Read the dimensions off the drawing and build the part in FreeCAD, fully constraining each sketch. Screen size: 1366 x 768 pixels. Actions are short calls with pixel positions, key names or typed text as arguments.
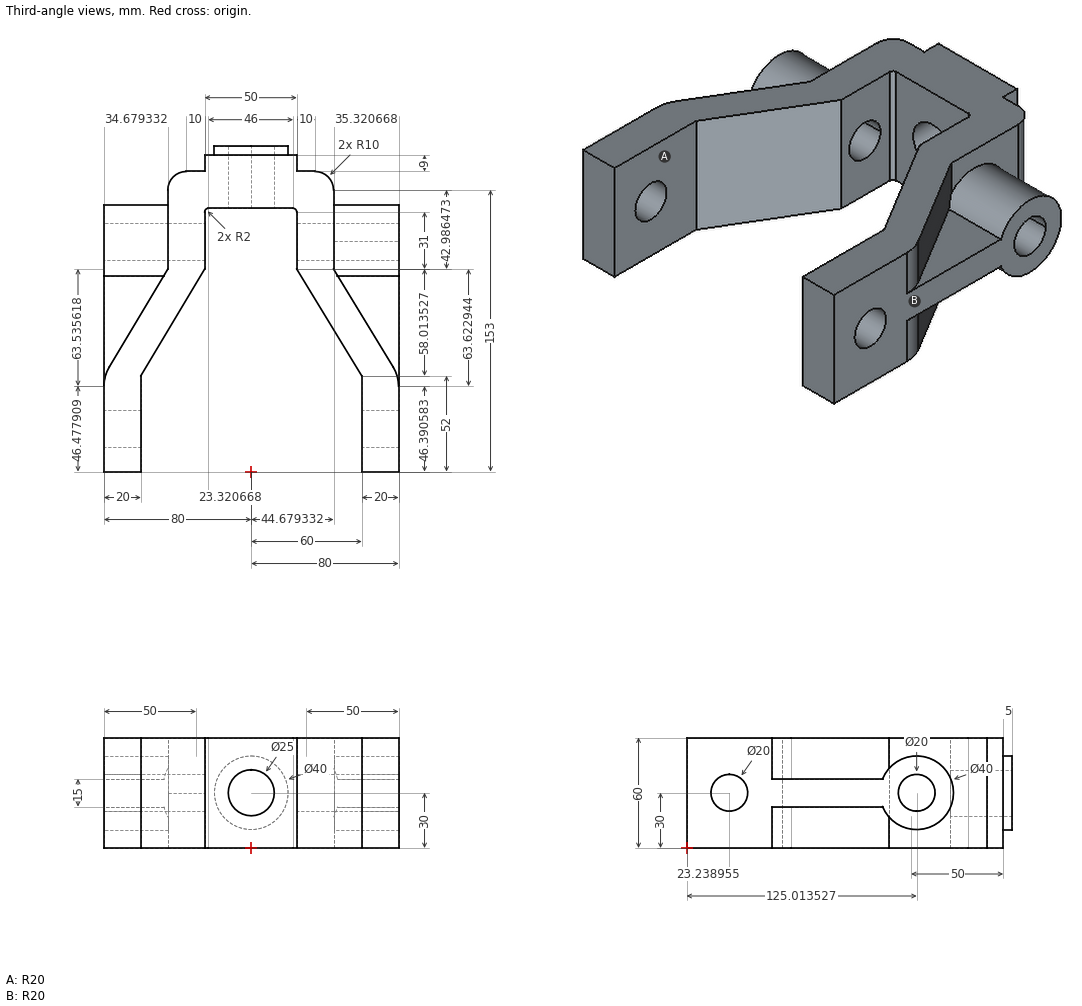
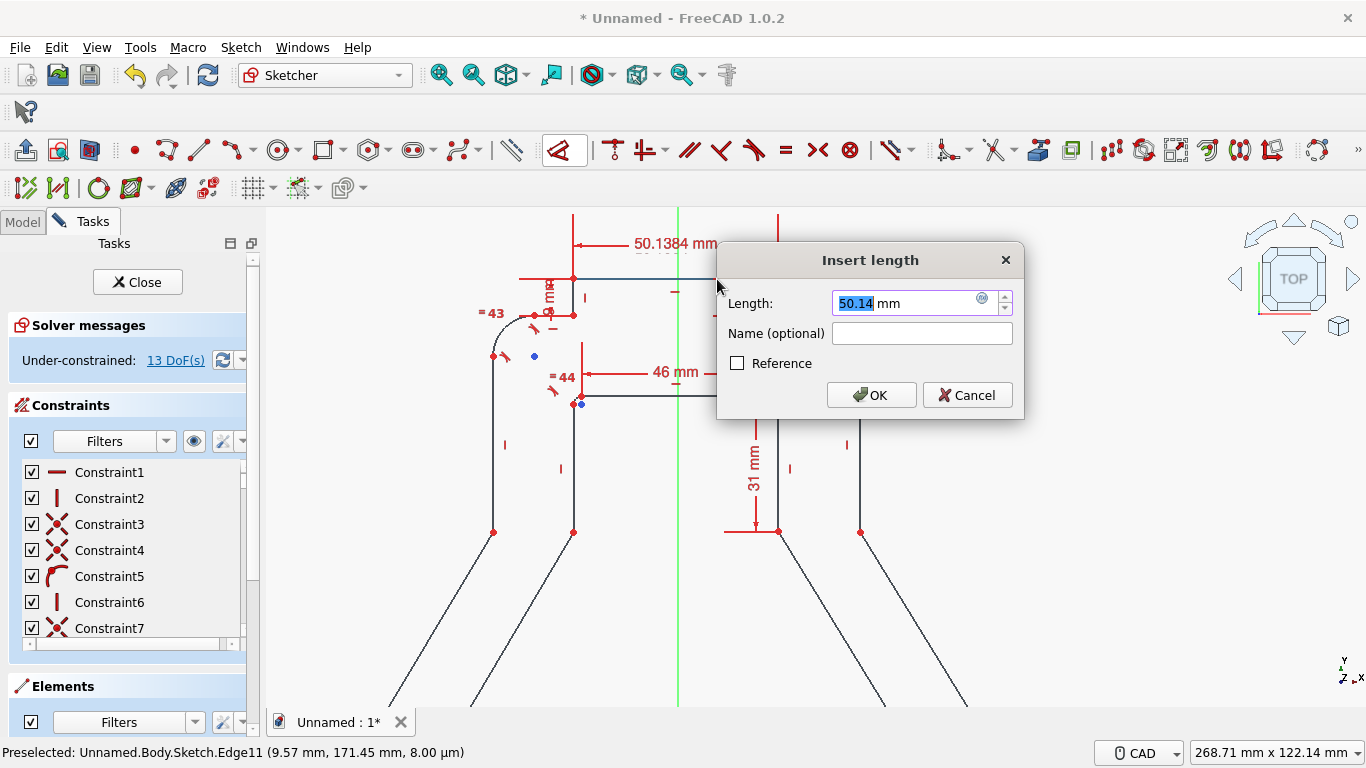
text(50)
key(Return)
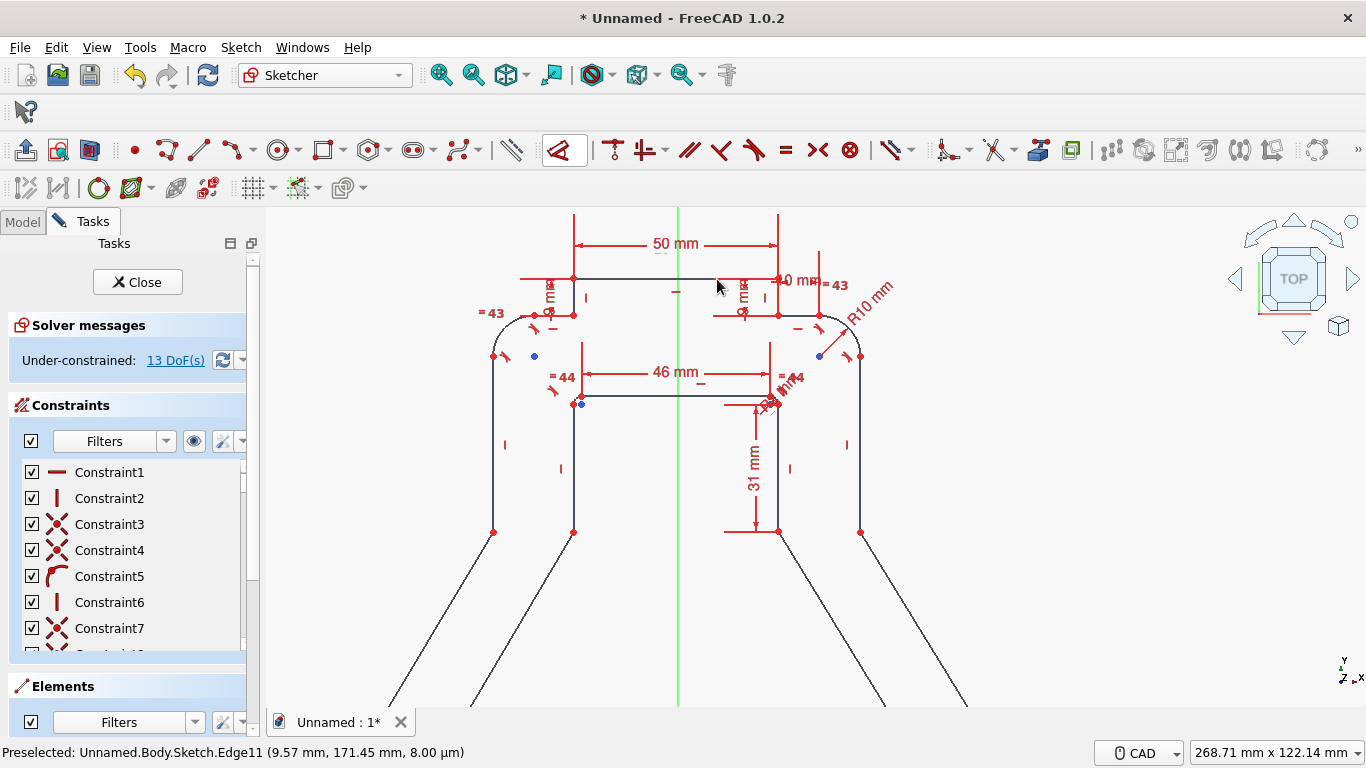
click(562, 316)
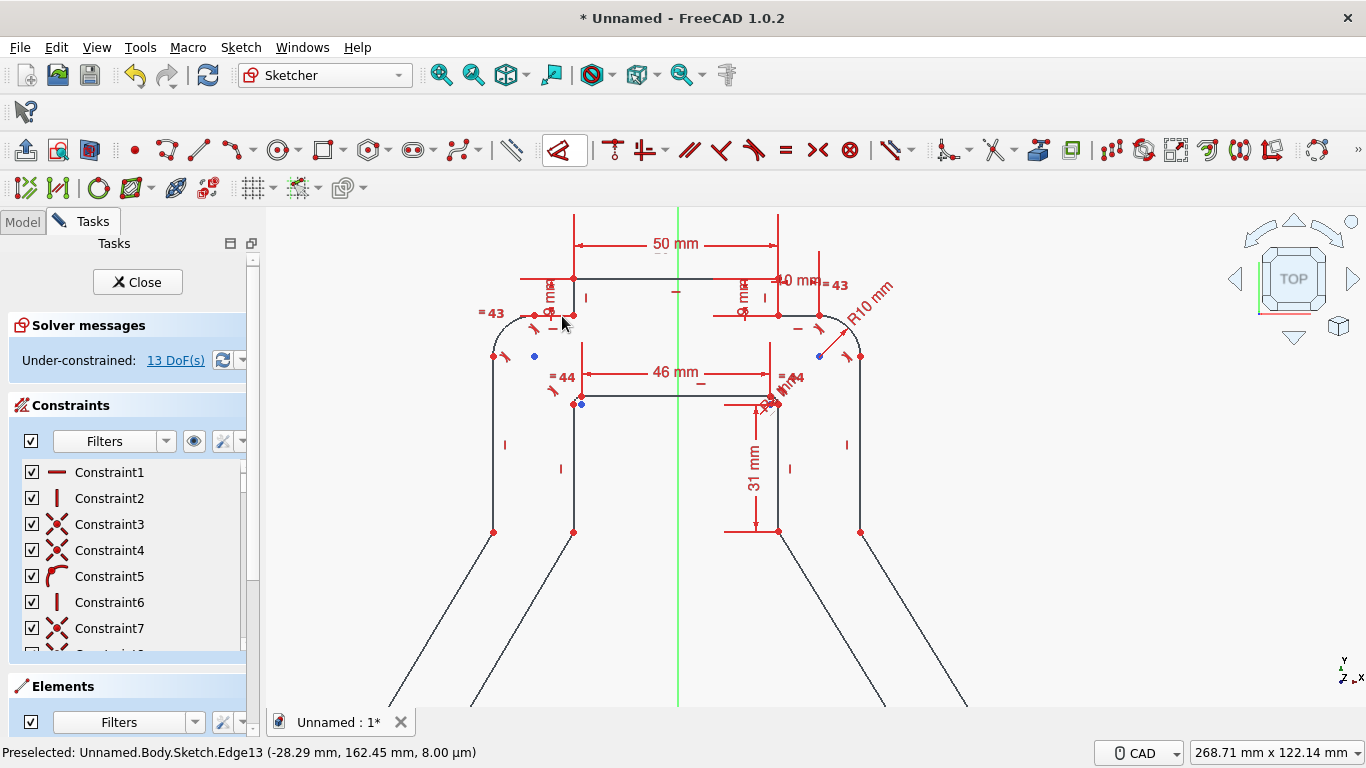
key(l)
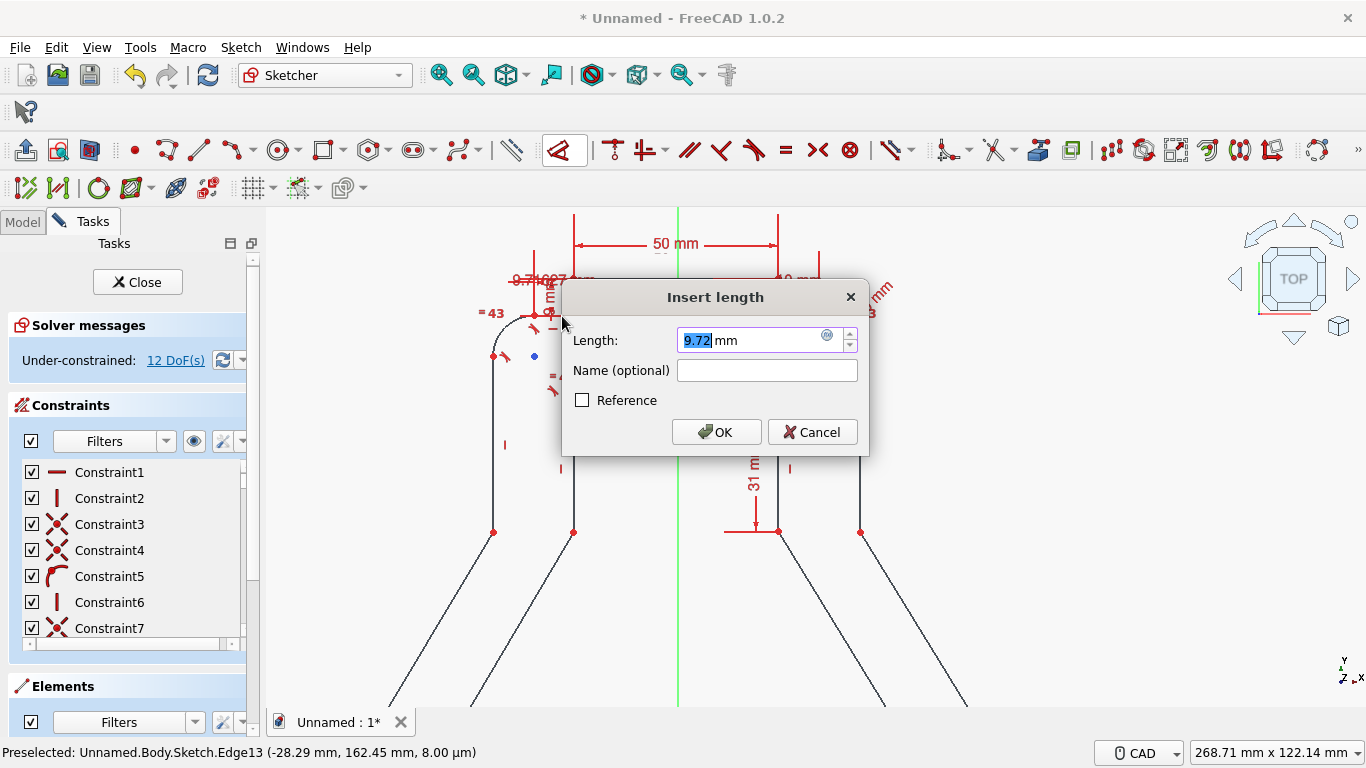
text(10)
key(Return)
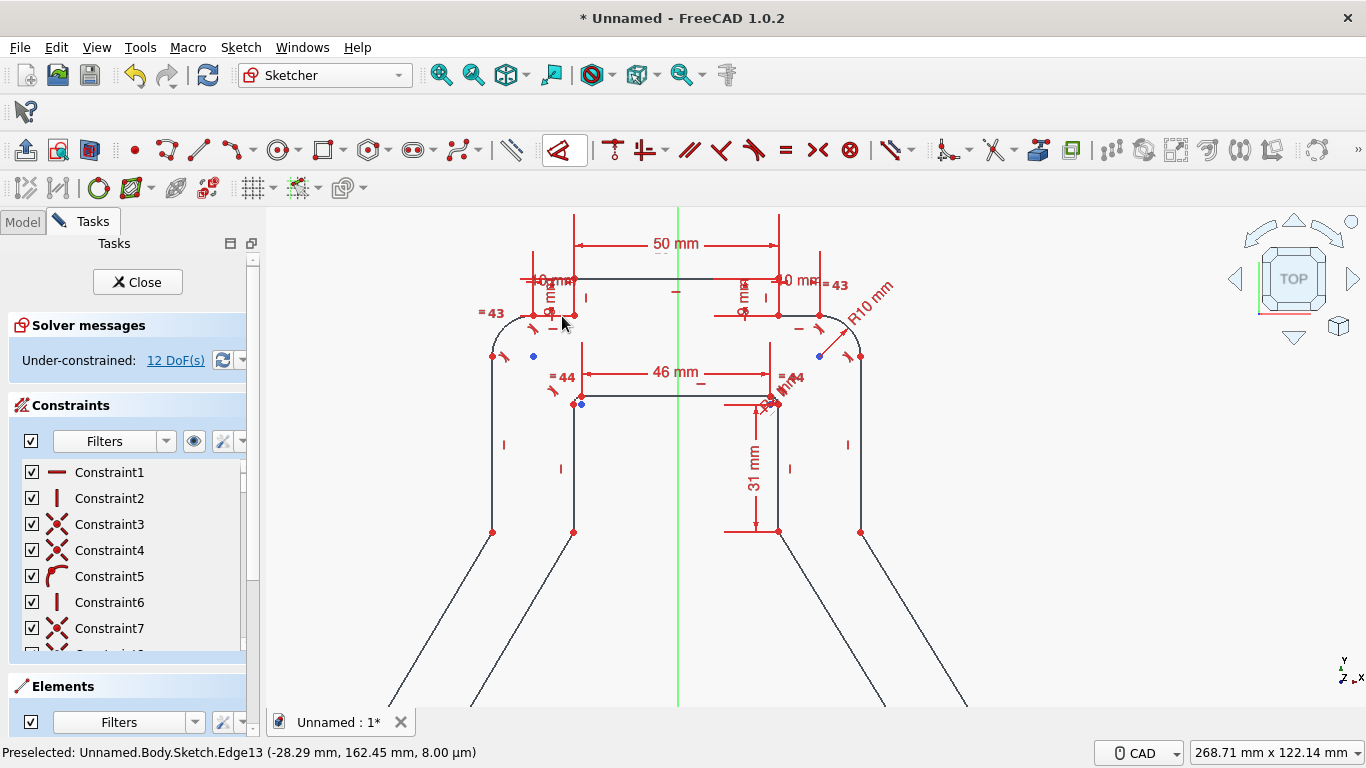
scroll(804, 317, down, 4)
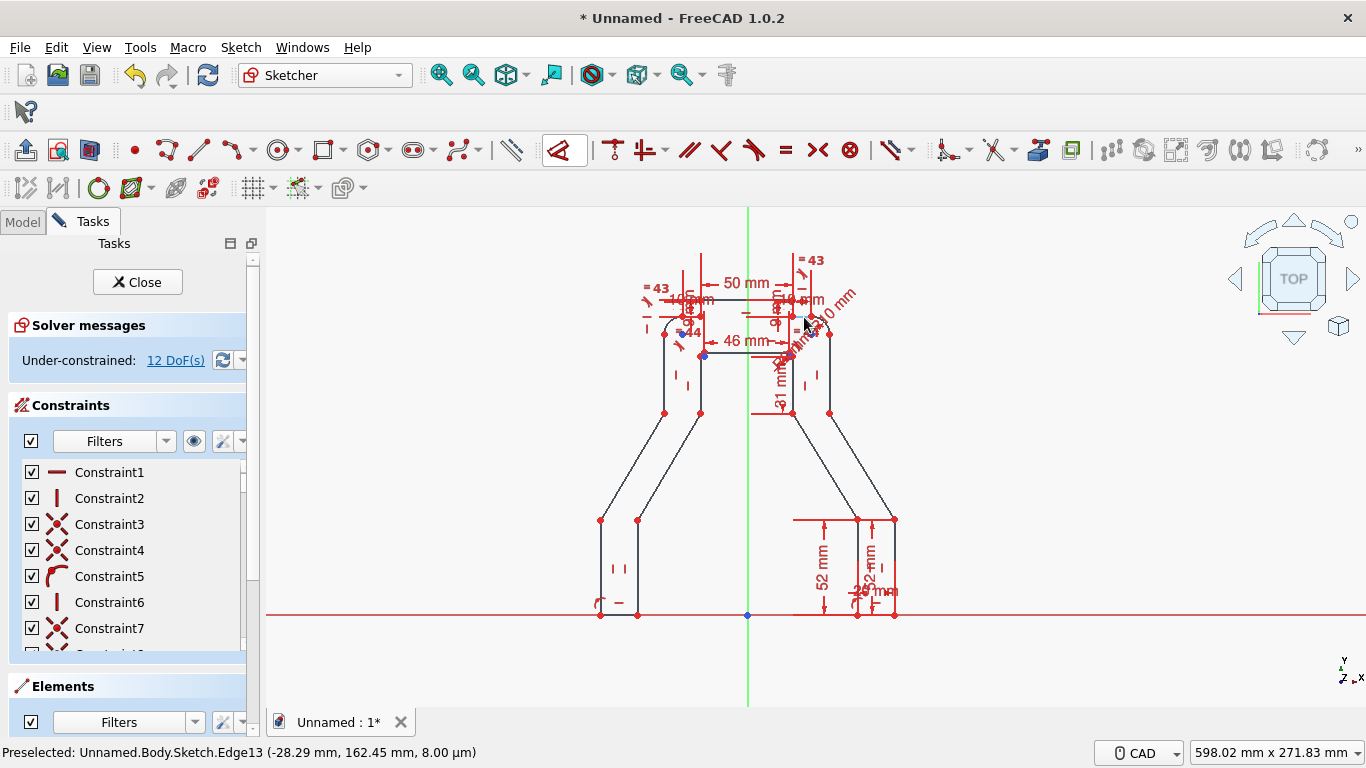
click(601, 549)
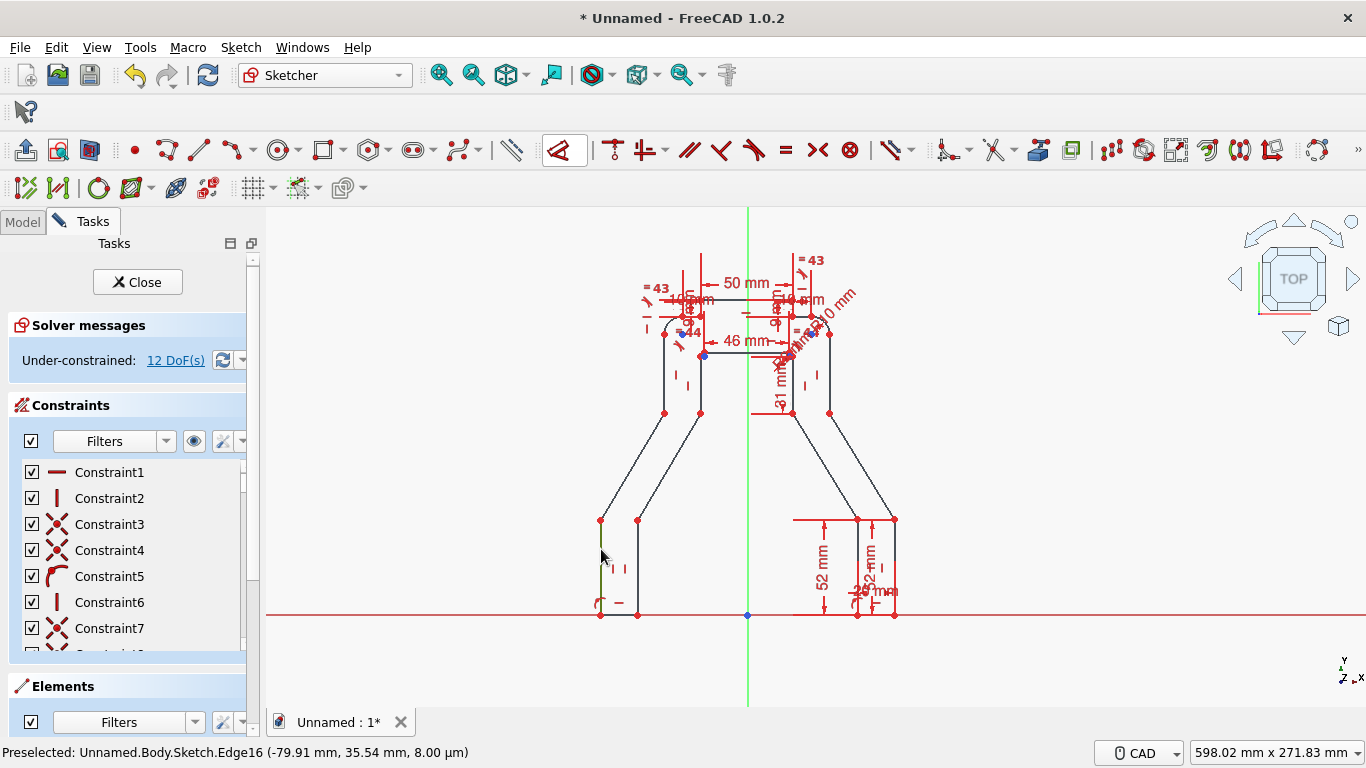
key(i)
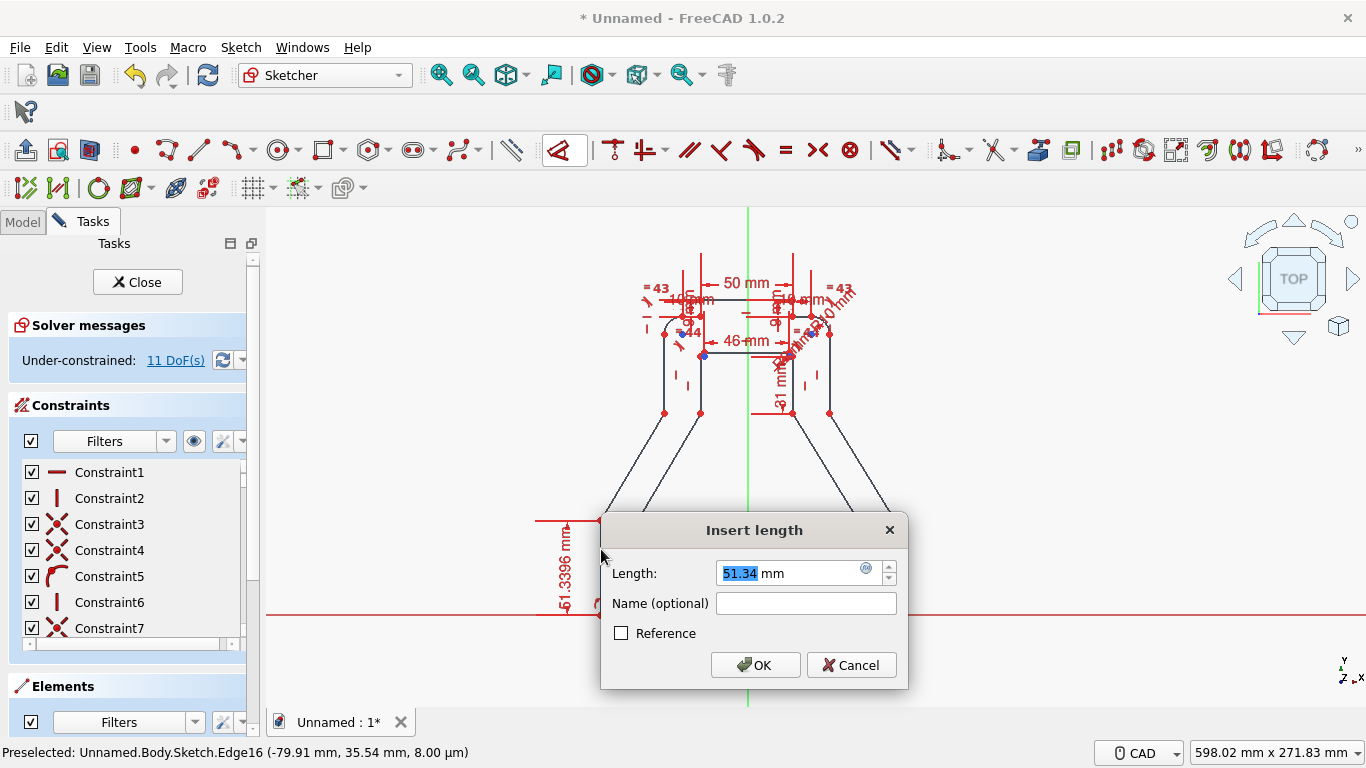
text(52)
key(Return)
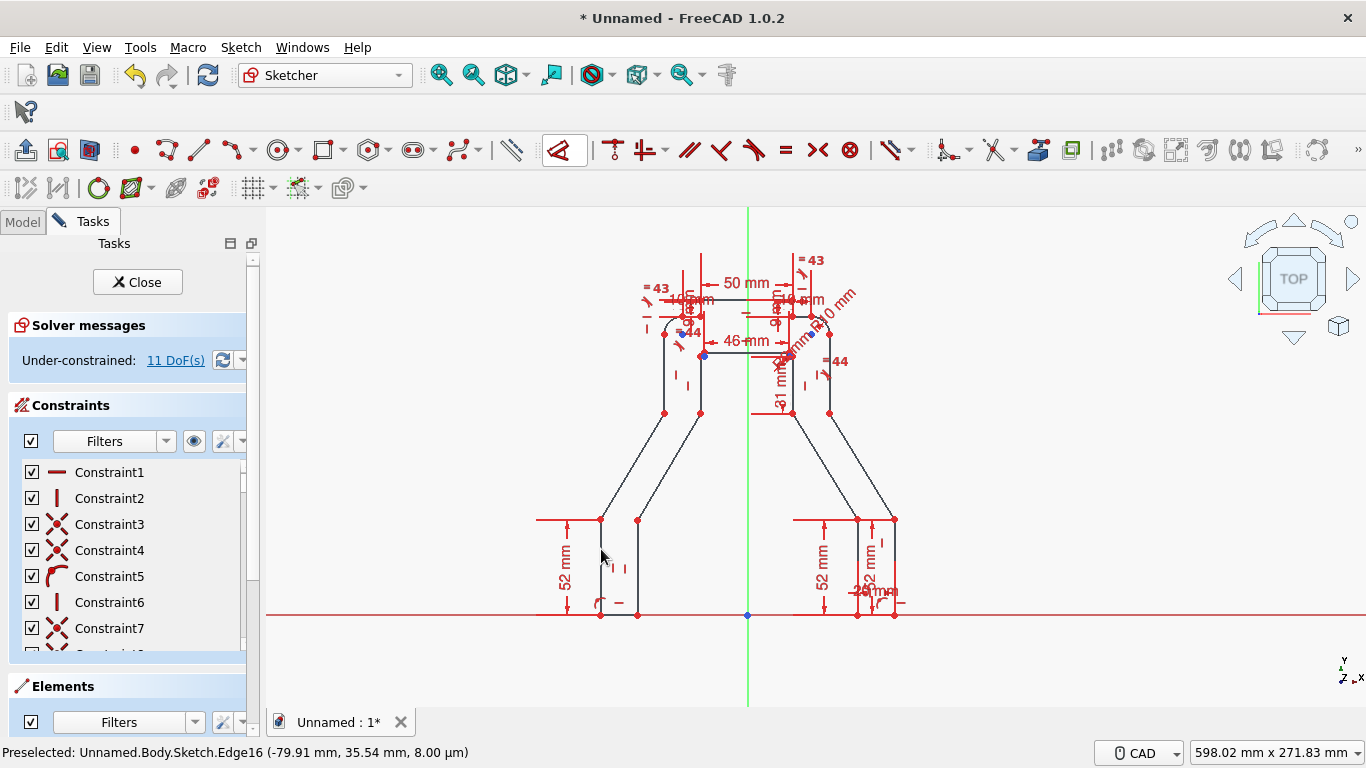
scroll(612, 615, up, 2)